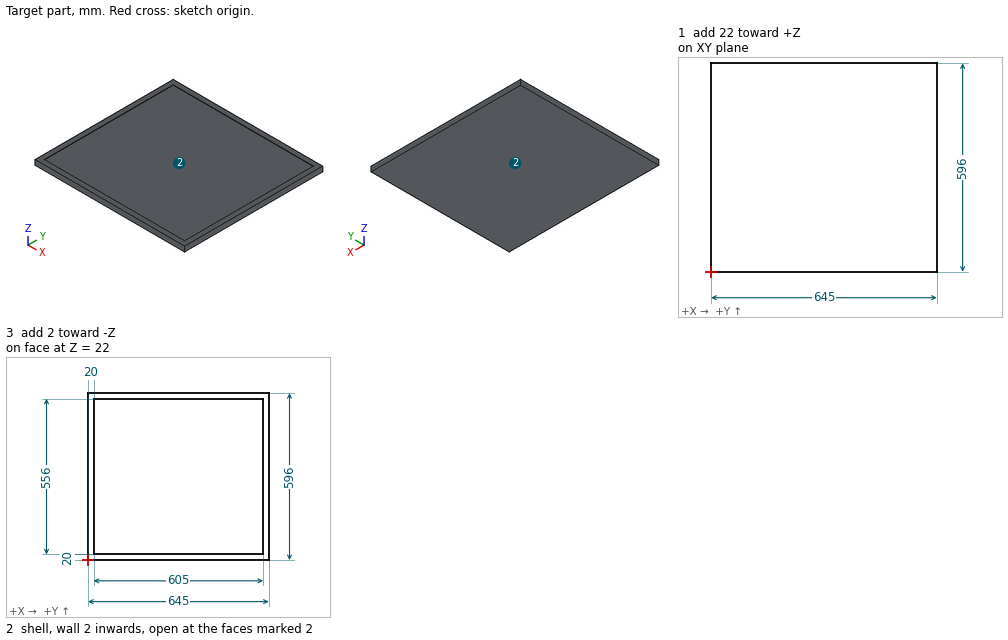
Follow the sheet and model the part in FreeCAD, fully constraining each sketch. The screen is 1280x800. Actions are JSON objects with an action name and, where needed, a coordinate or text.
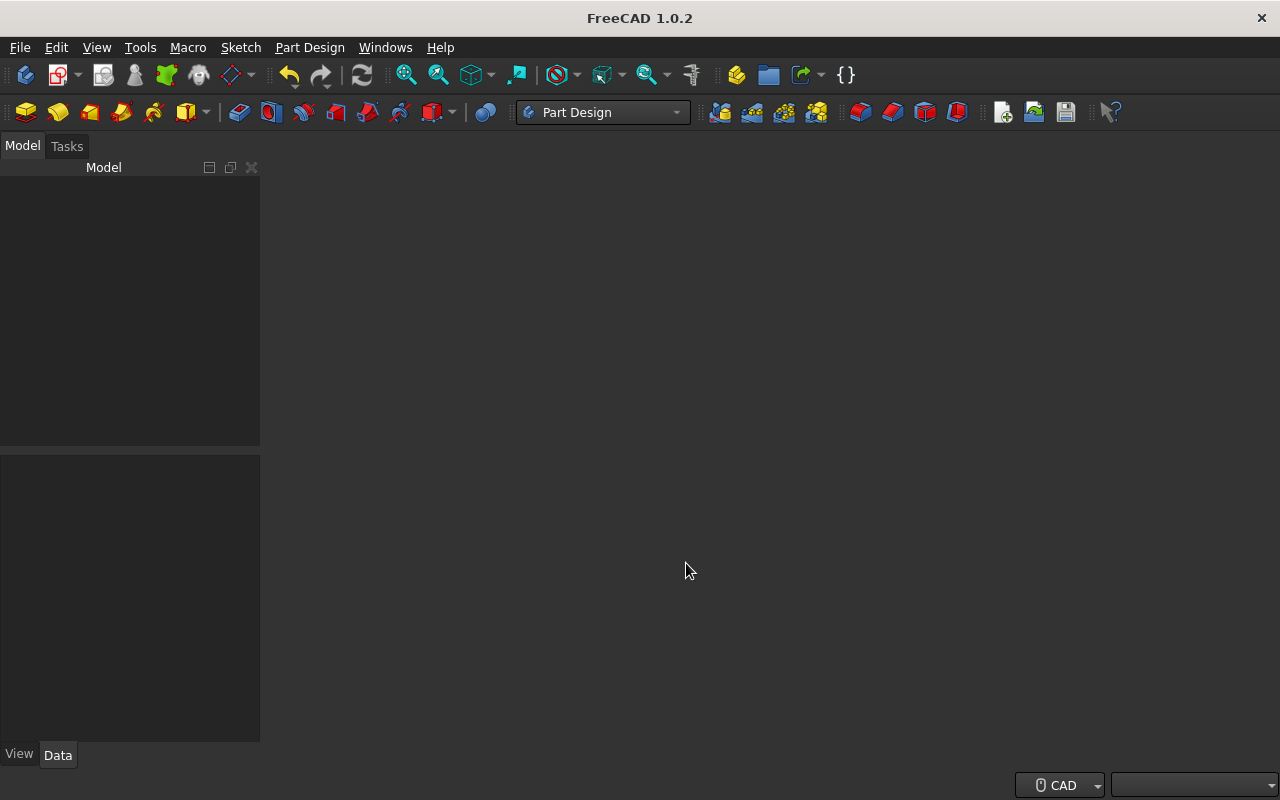
{"action": "key", "text": "ctrl+n"}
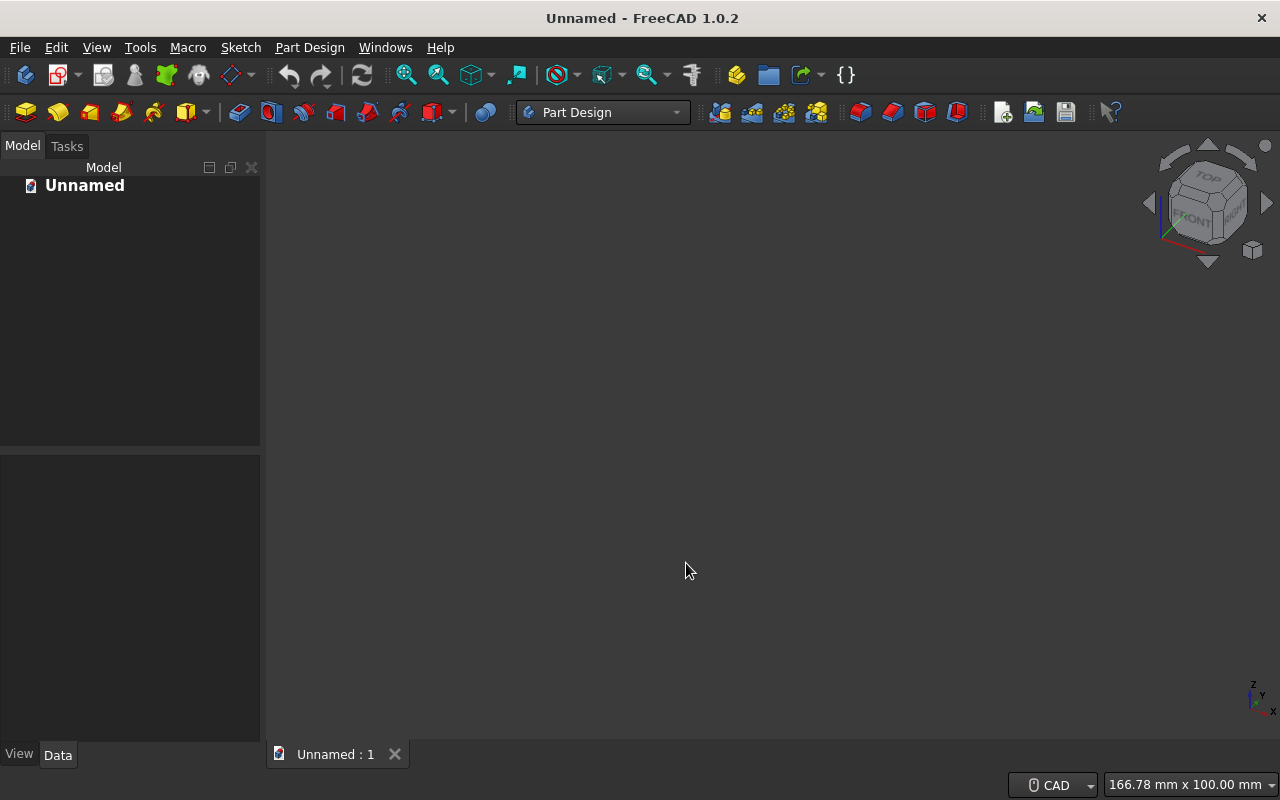
{"action": "left_click", "coordinate": [58, 76]}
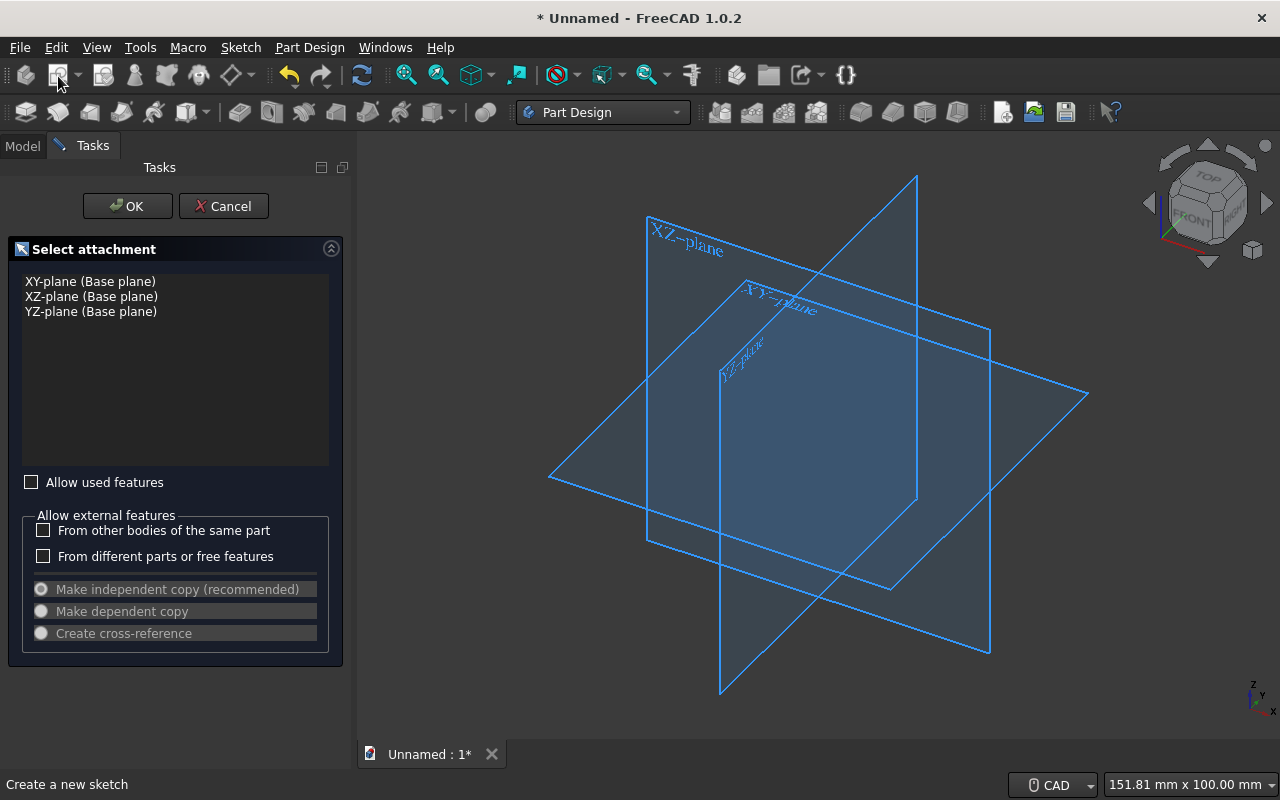
{"action": "left_click", "coordinate": [82, 282]}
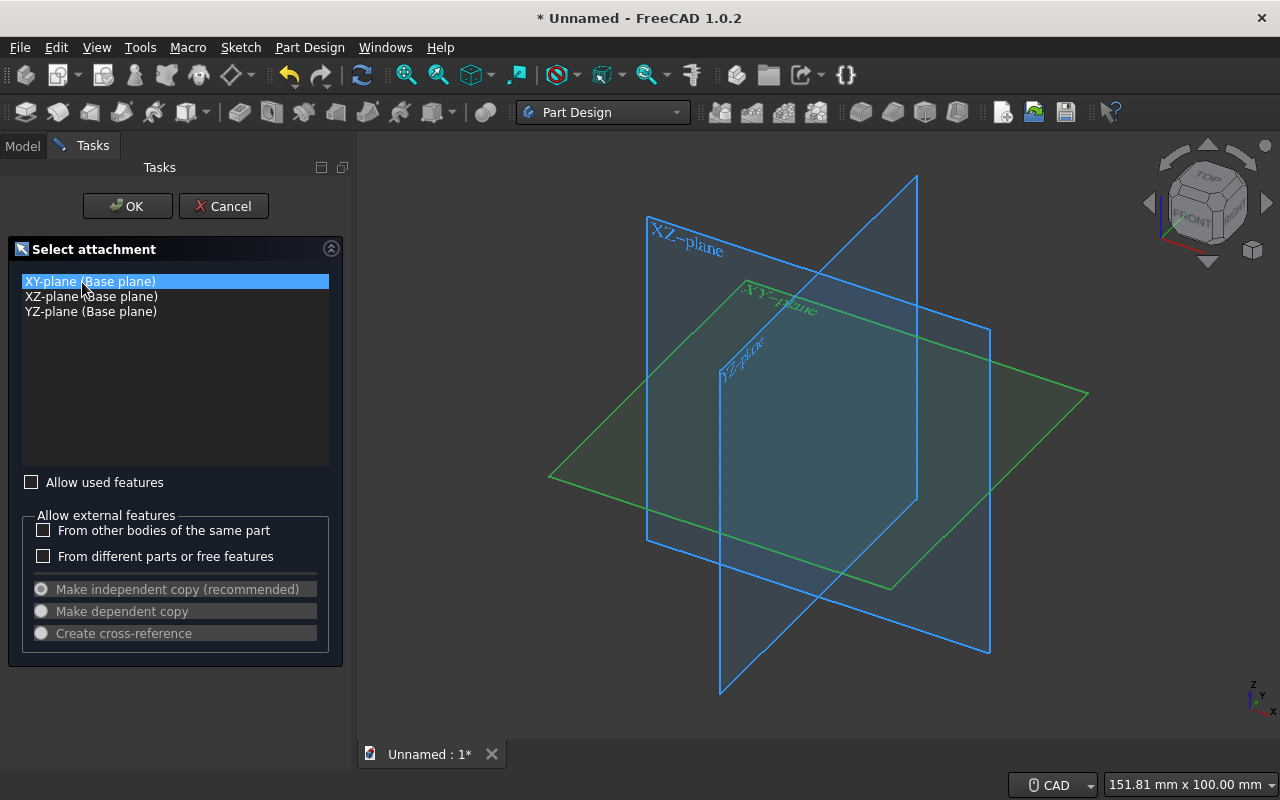
{"action": "left_click", "coordinate": [128, 206]}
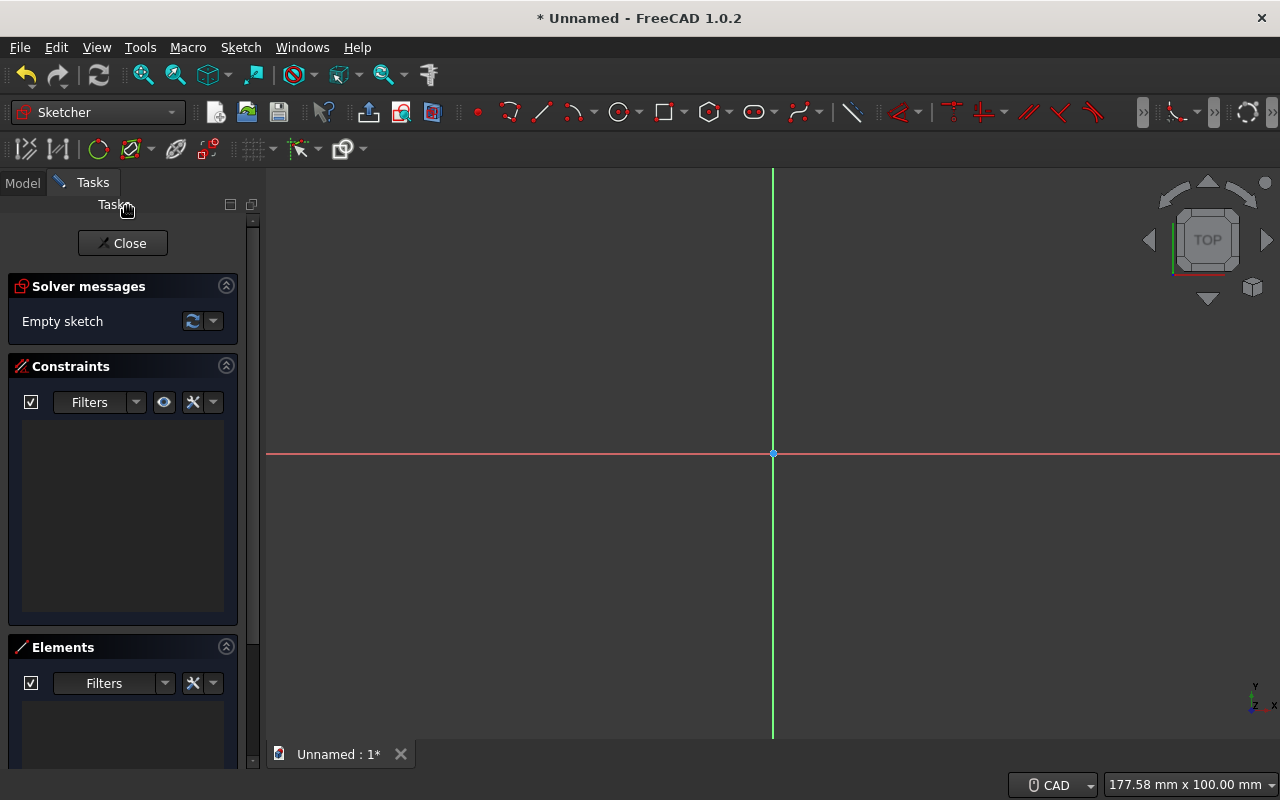
{"action": "scroll", "coordinate": [466, 666], "scroll_direction": "down", "scroll_amount": 11}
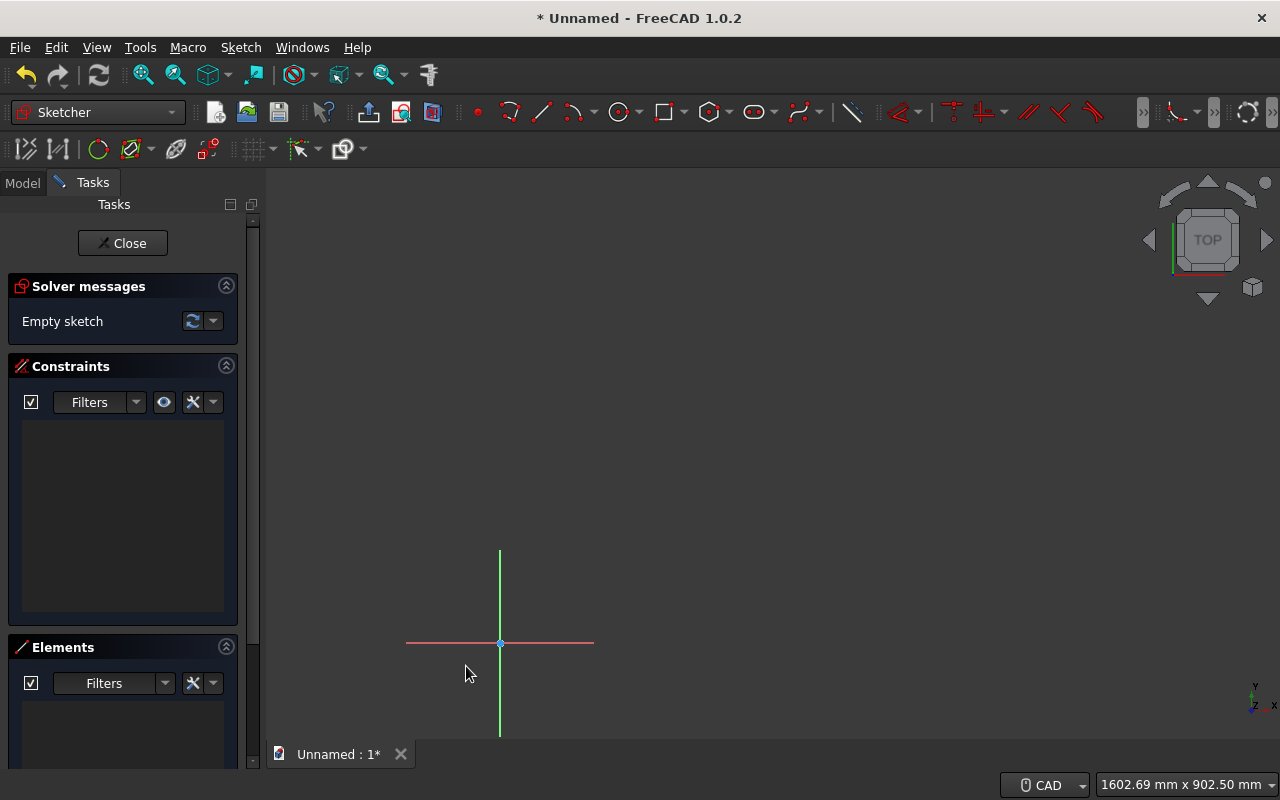
{"action": "left_click", "coordinate": [664, 112]}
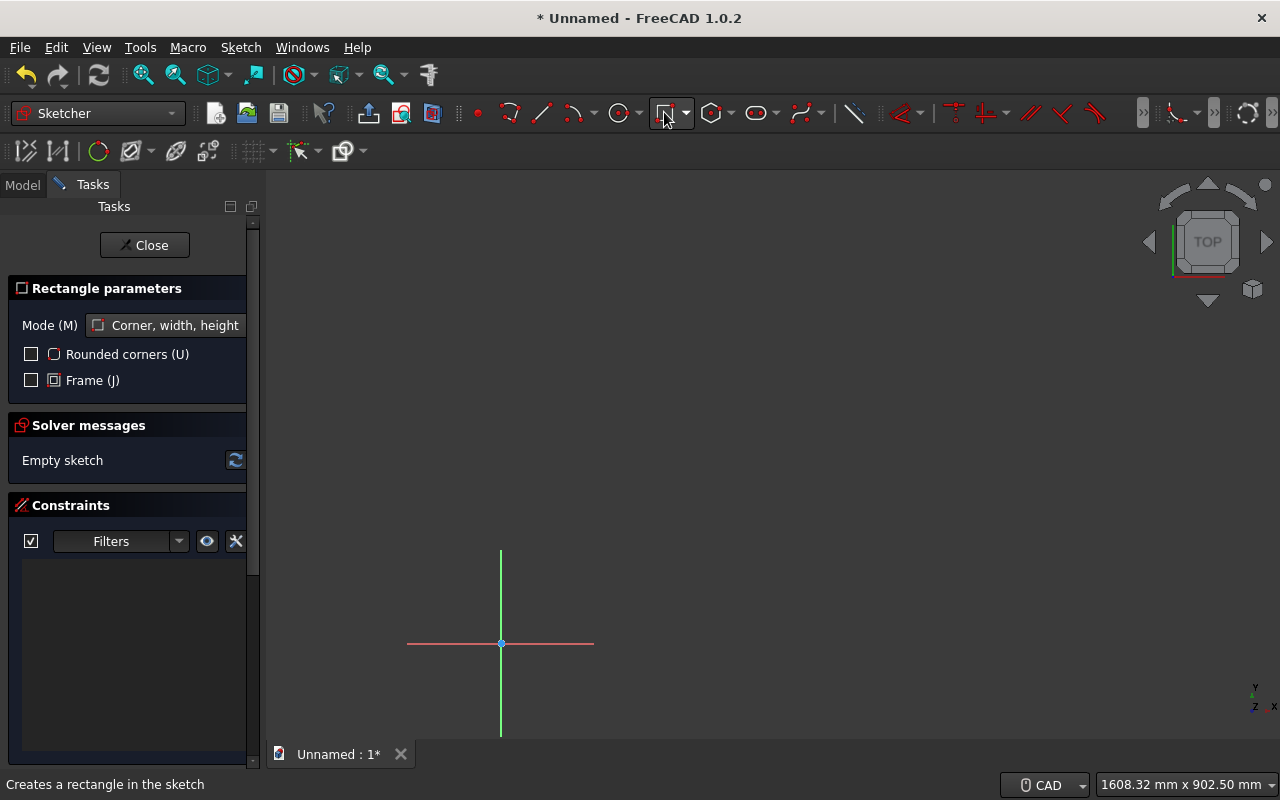
{"action": "left_click", "coordinate": [501, 644]}
{"action": "left_click", "coordinate": [908, 268]}
{"action": "key", "text": "Escape"}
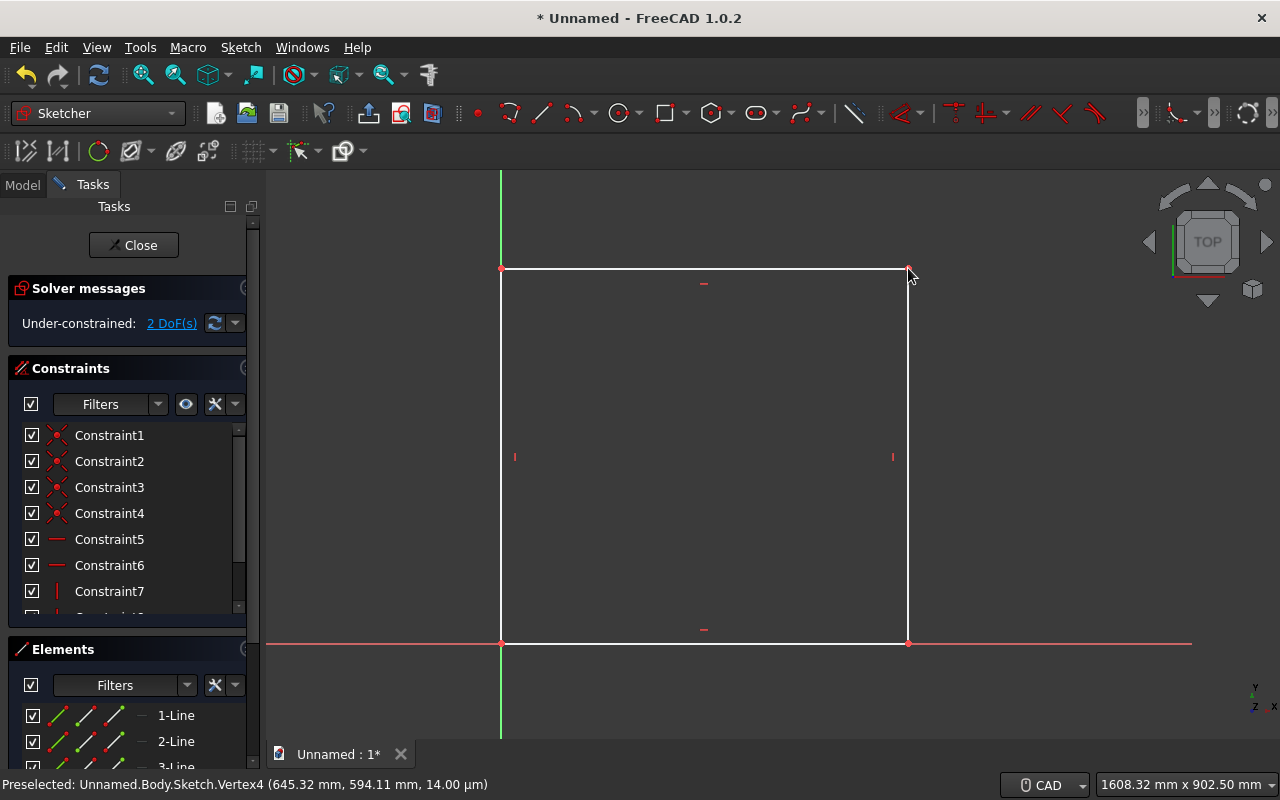
{"action": "left_click", "coordinate": [623, 644]}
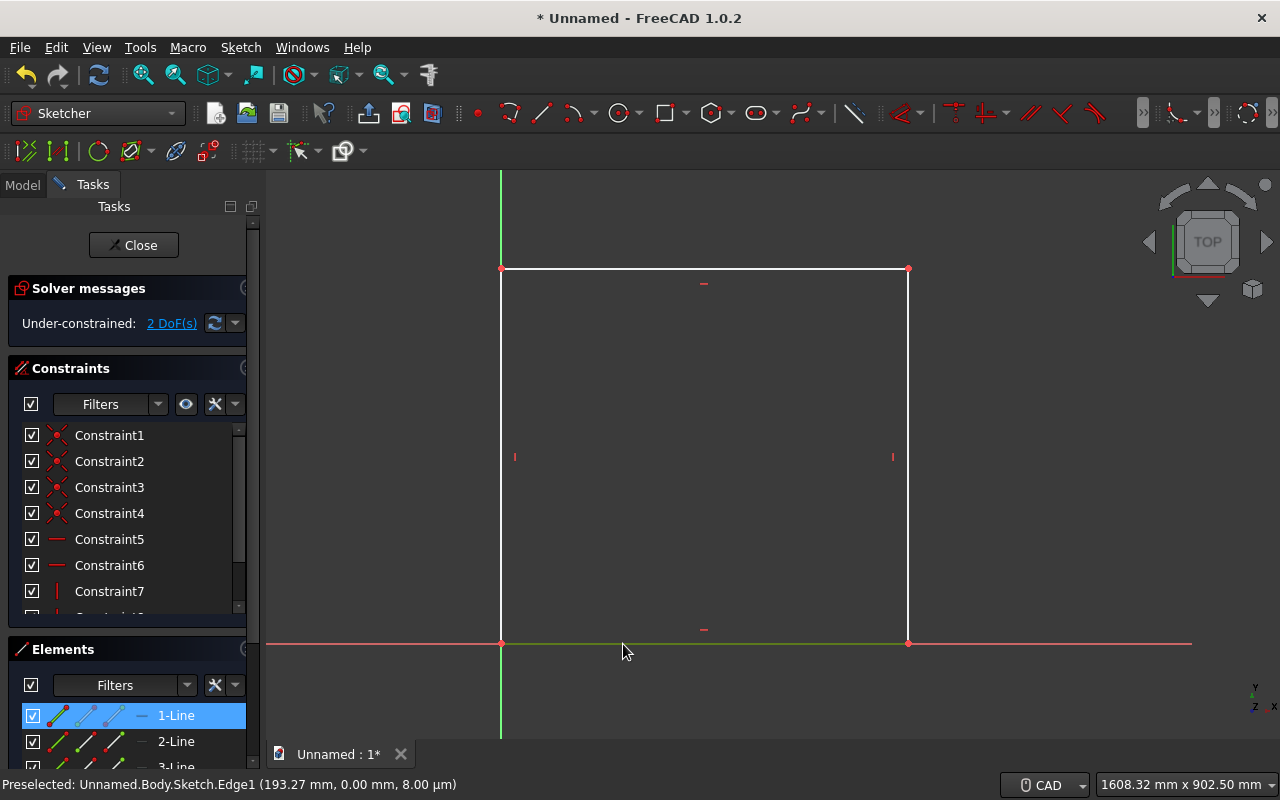
{"action": "left_click", "coordinate": [922, 114]}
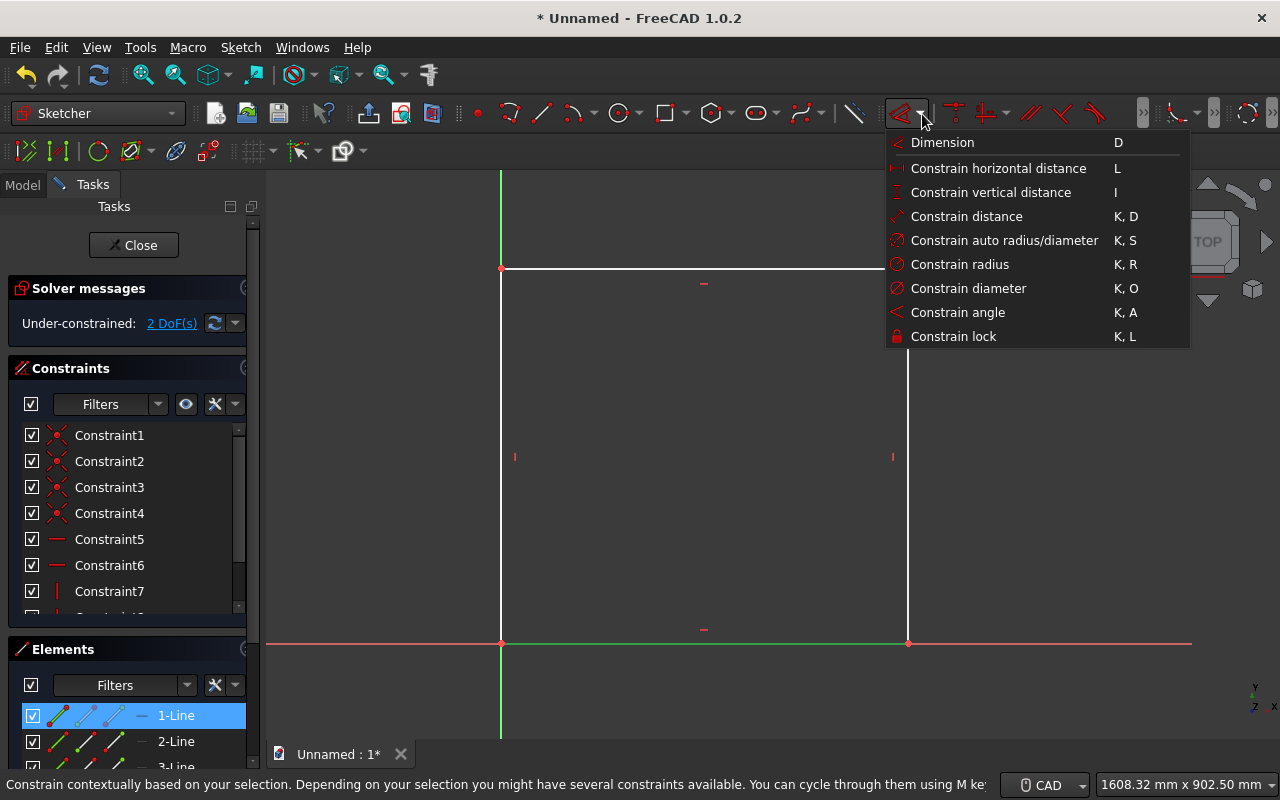
{"action": "left_click", "coordinate": [1038, 168]}